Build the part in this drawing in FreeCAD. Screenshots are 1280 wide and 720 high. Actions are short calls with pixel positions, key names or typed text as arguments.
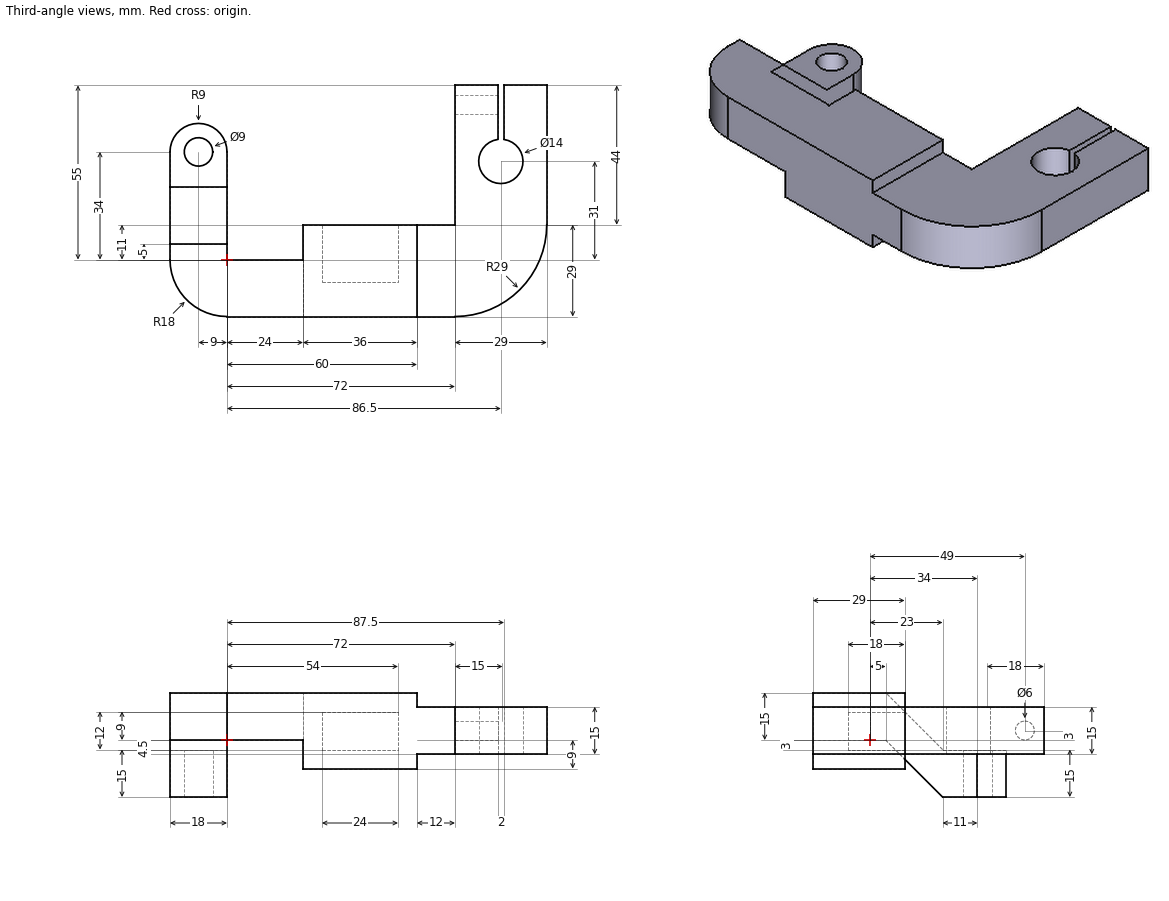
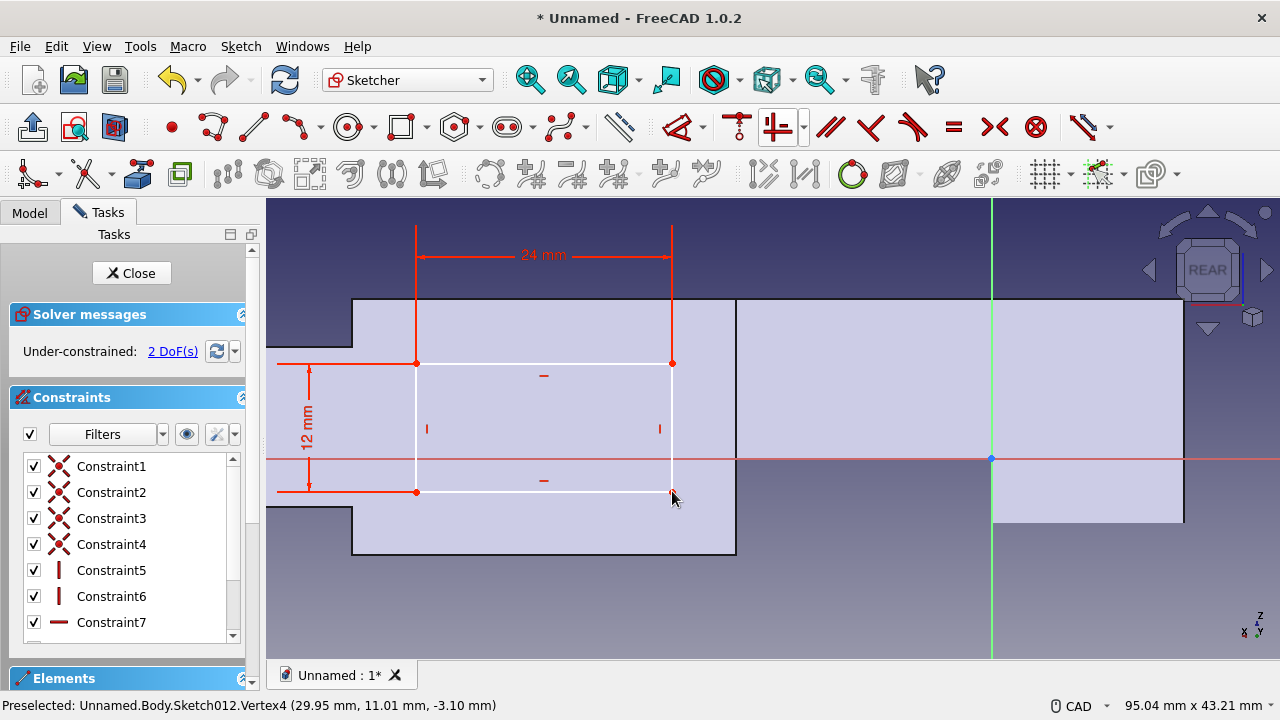
click(676, 128)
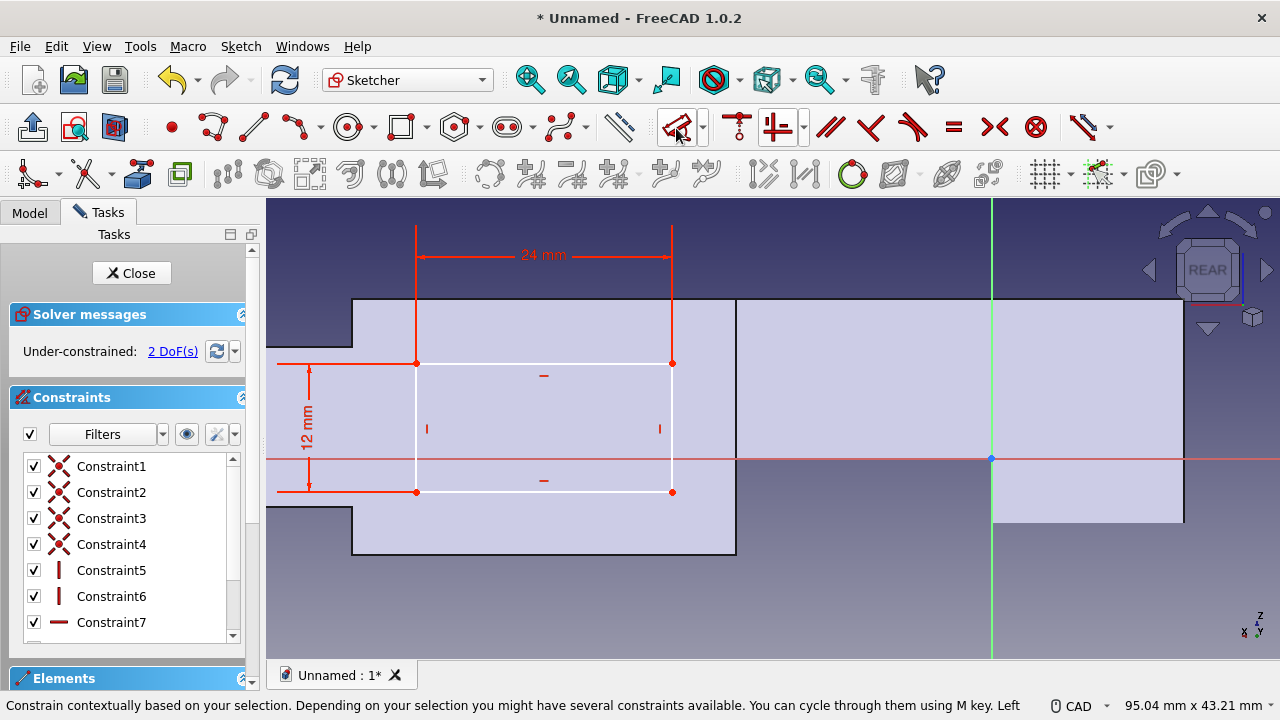
click(416, 364)
click(1026, 411)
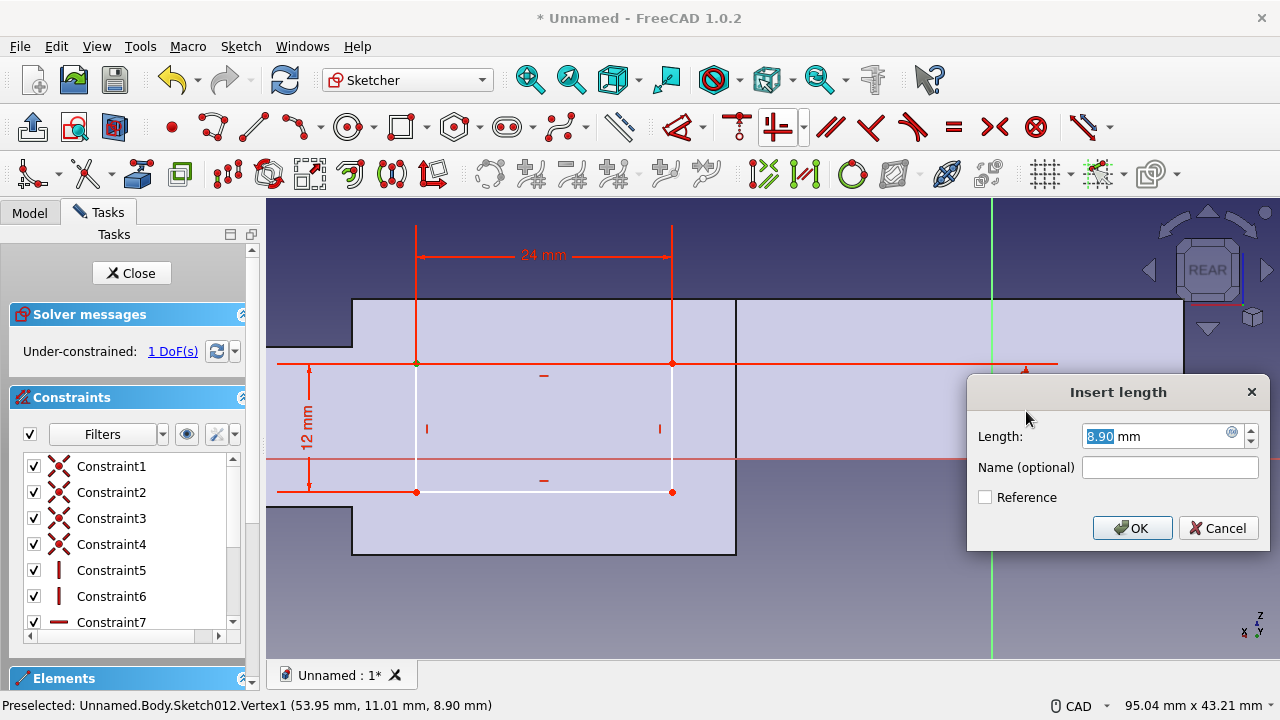
text(9)
key(Return)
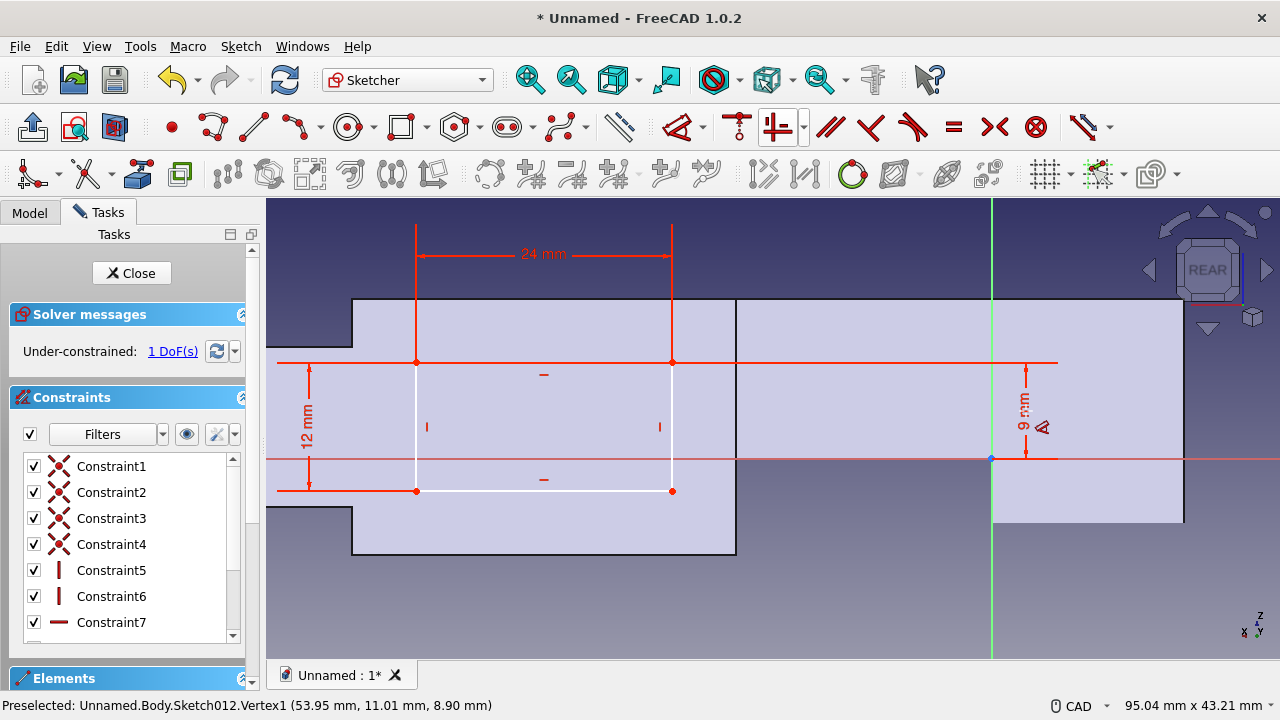
click(416, 363)
click(704, 329)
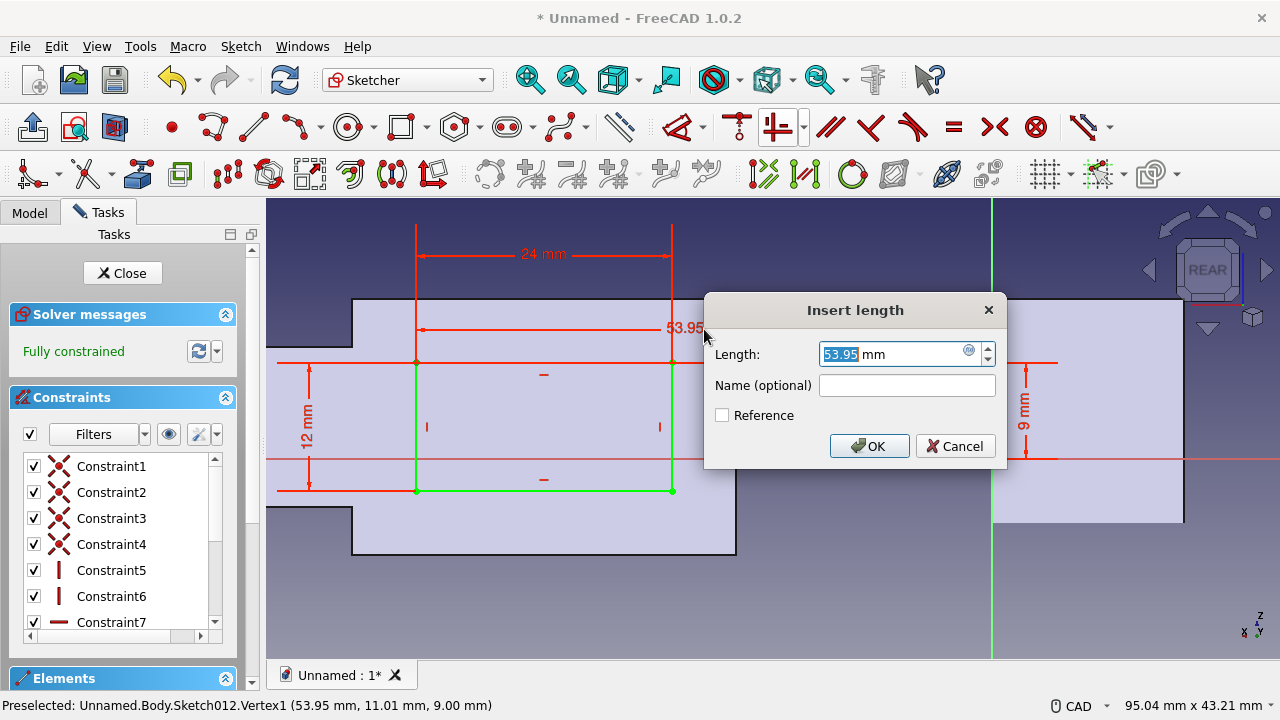
text(54)
key(Return)
key(Escape)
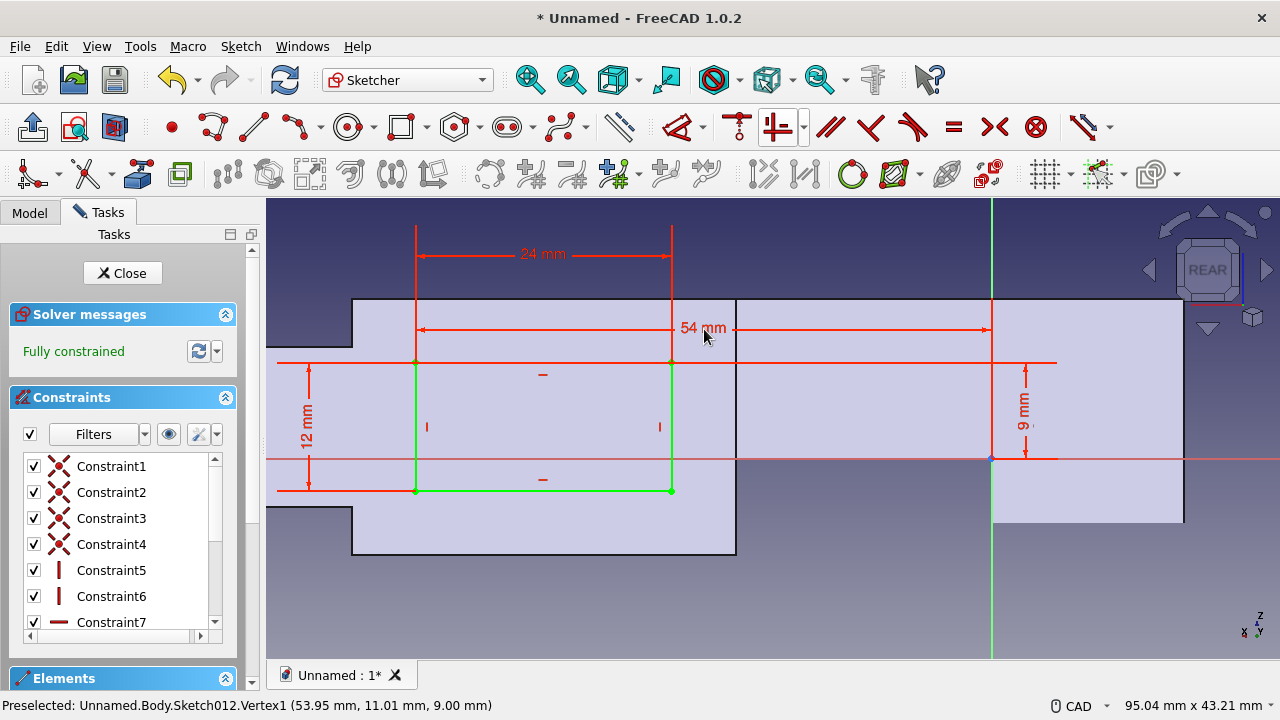
click(123, 273)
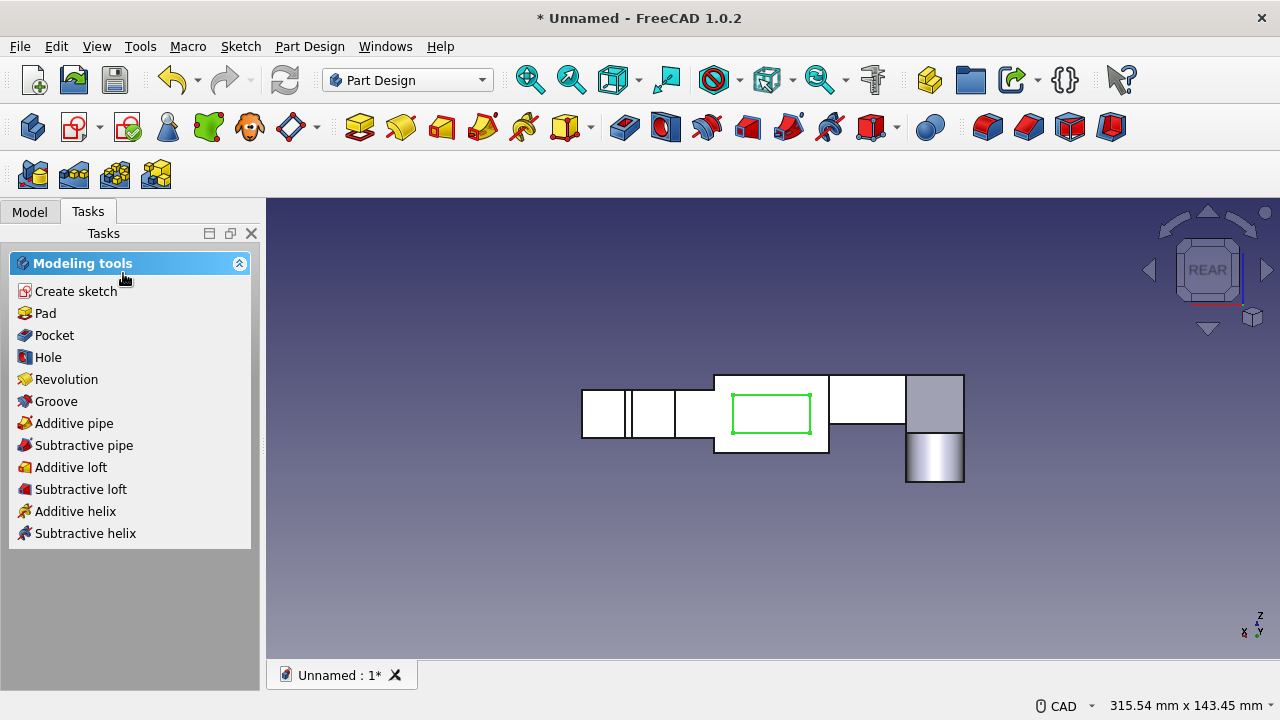
click(625, 128)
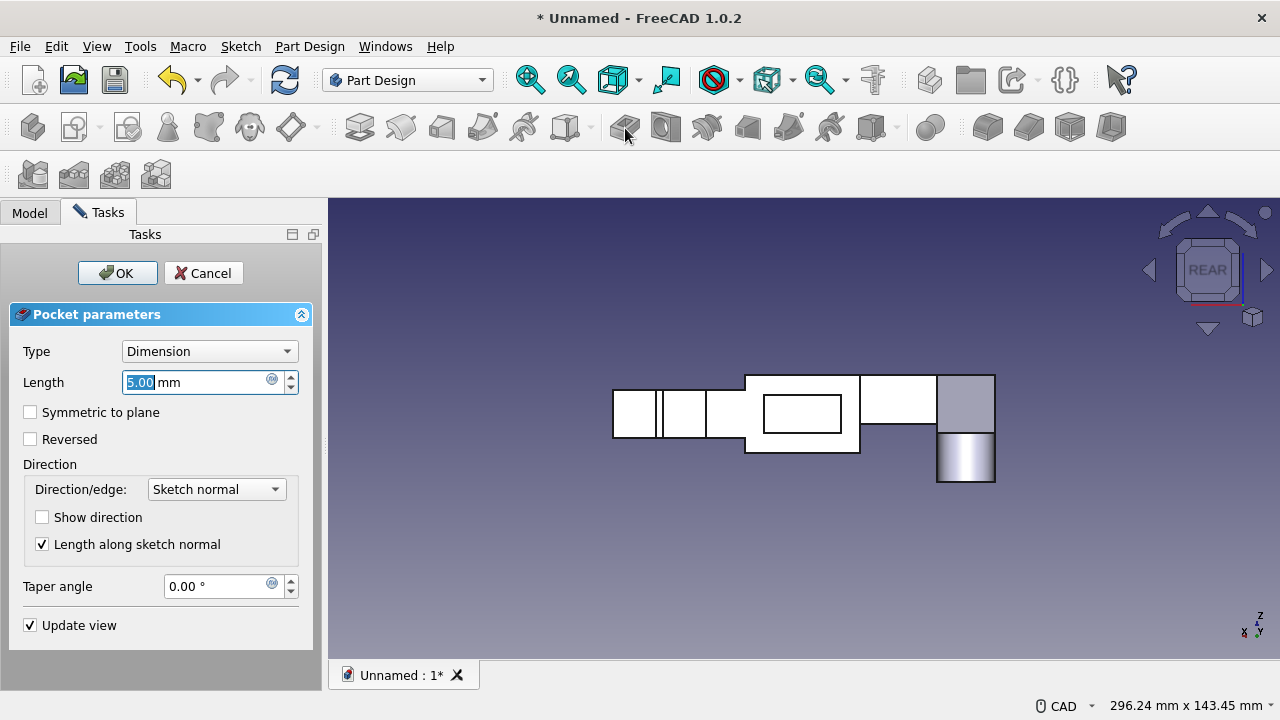
text(18)
key(Tab)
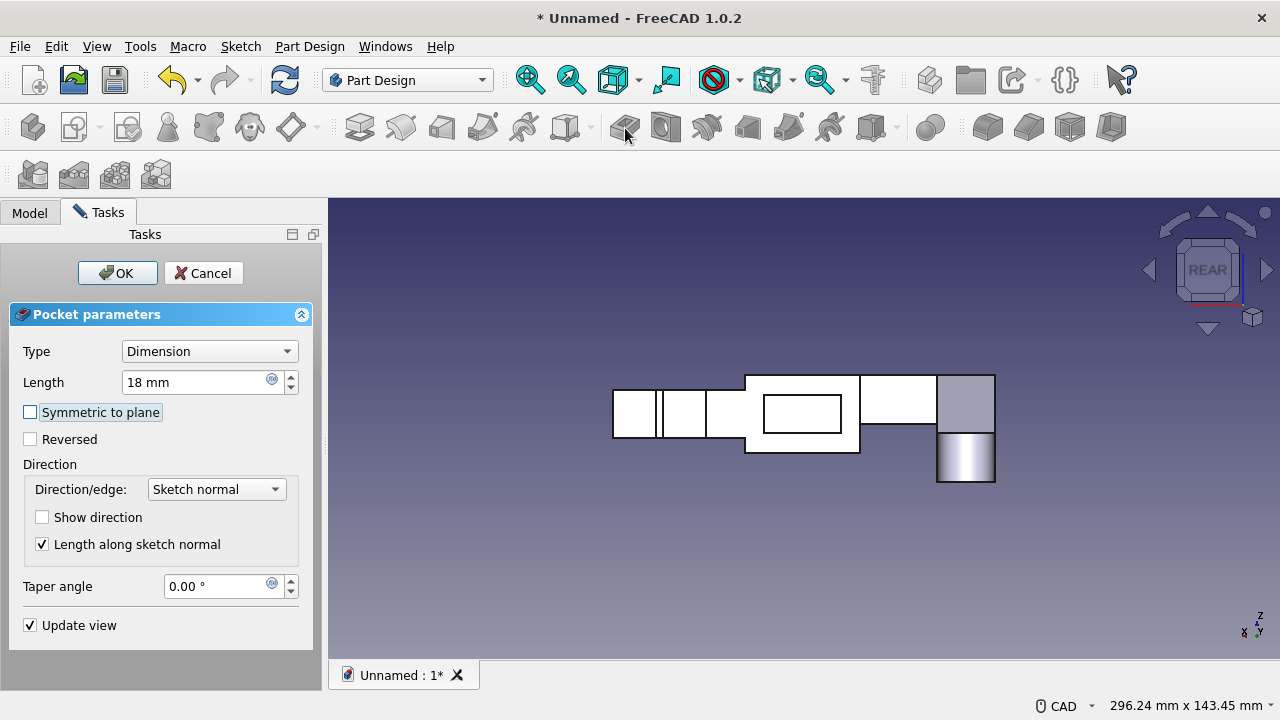
click(118, 273)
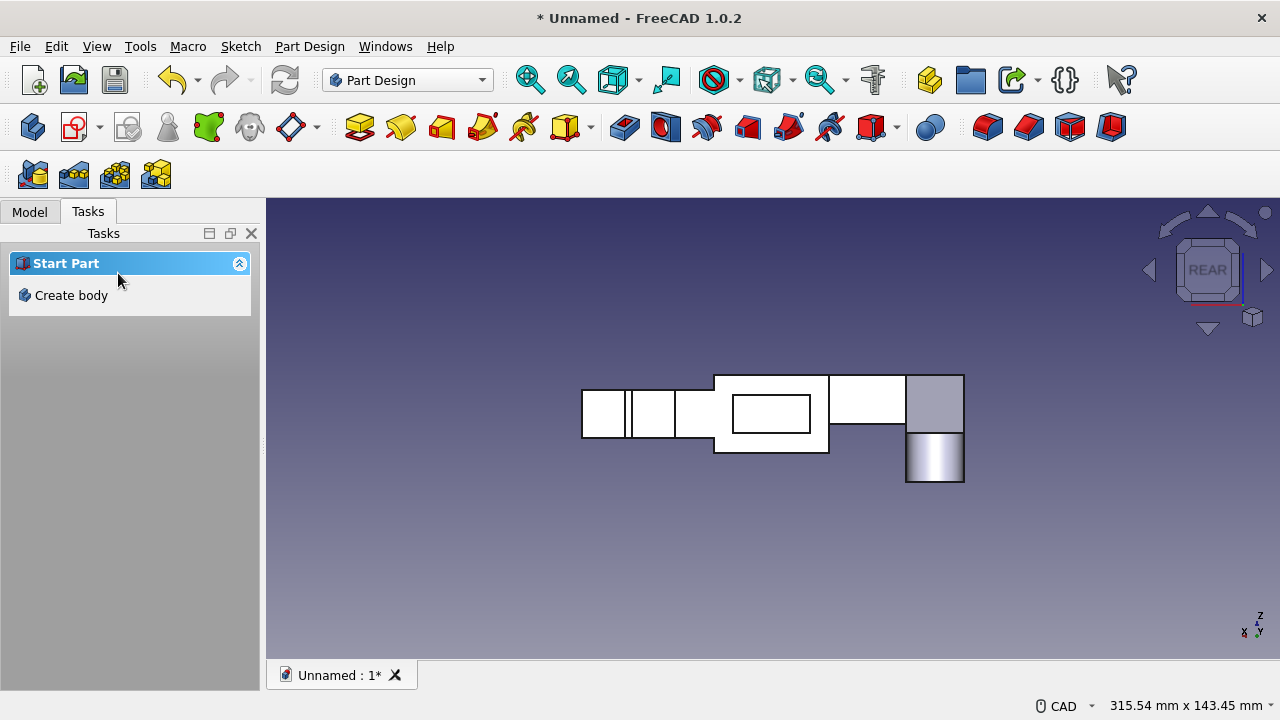
key(0)